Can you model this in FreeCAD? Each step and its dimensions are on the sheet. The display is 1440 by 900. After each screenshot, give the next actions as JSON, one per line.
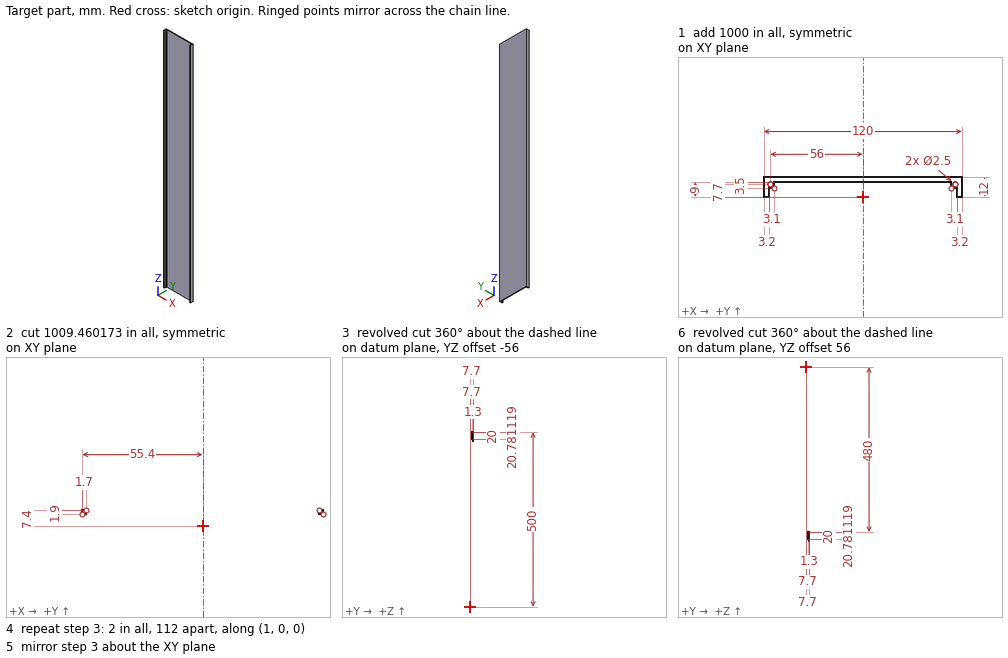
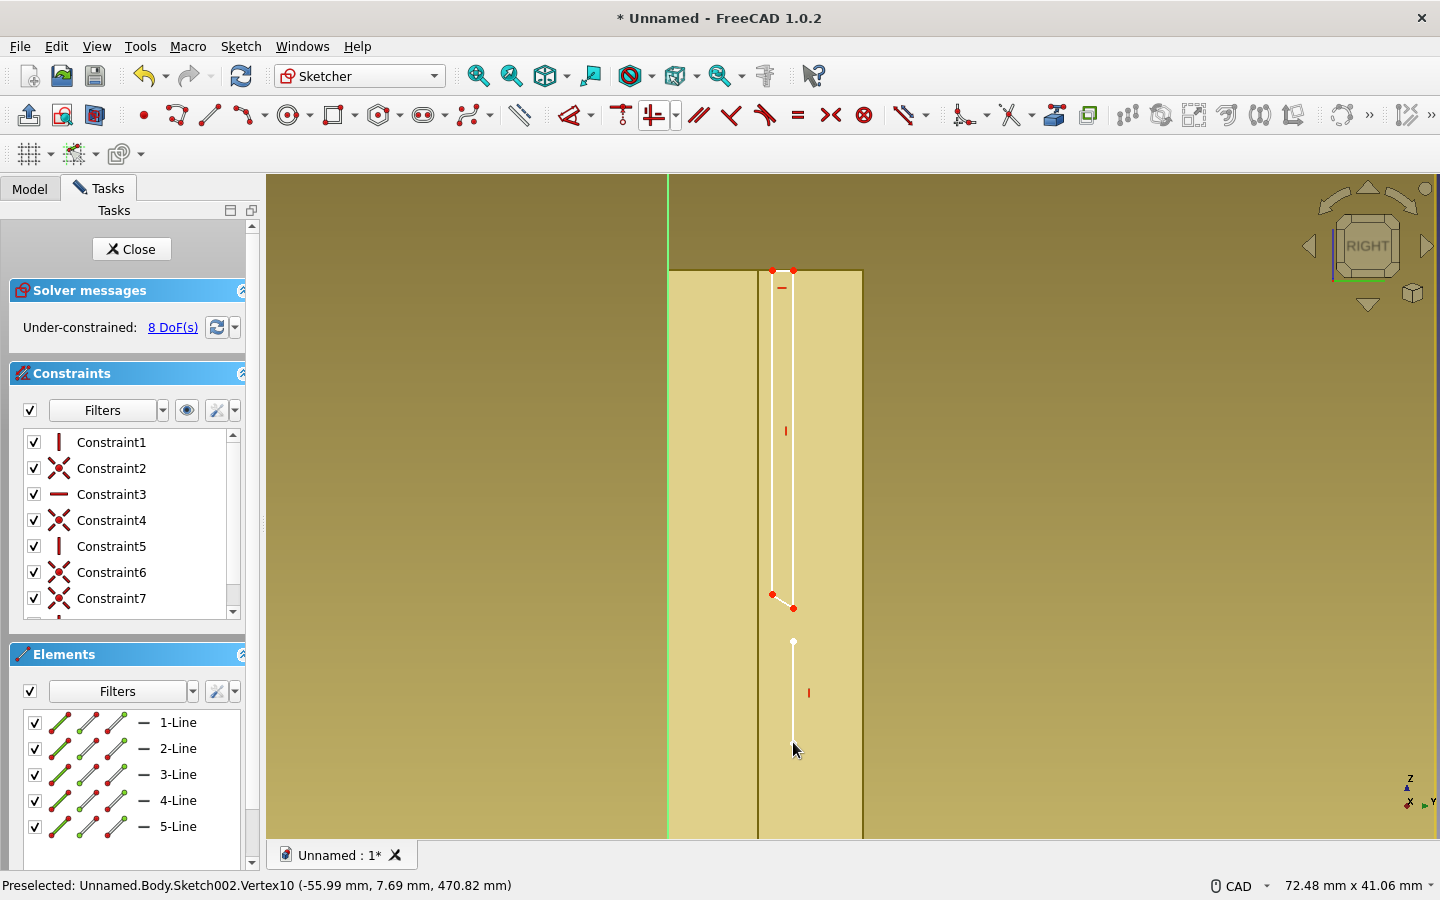
{"action": "left_click", "coordinate": [793, 672]}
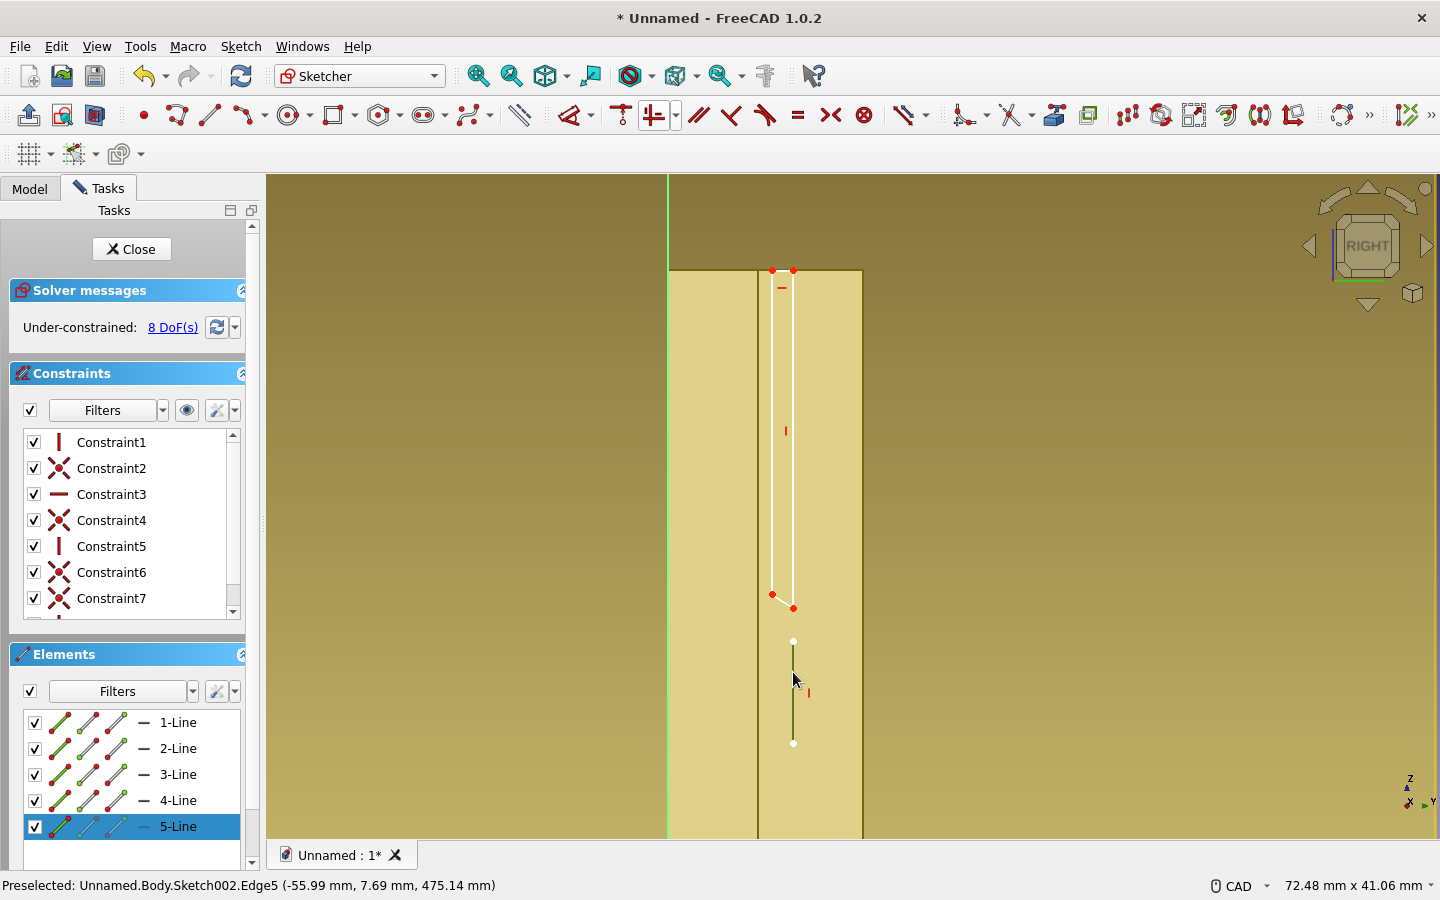
{"action": "key", "text": "g n"}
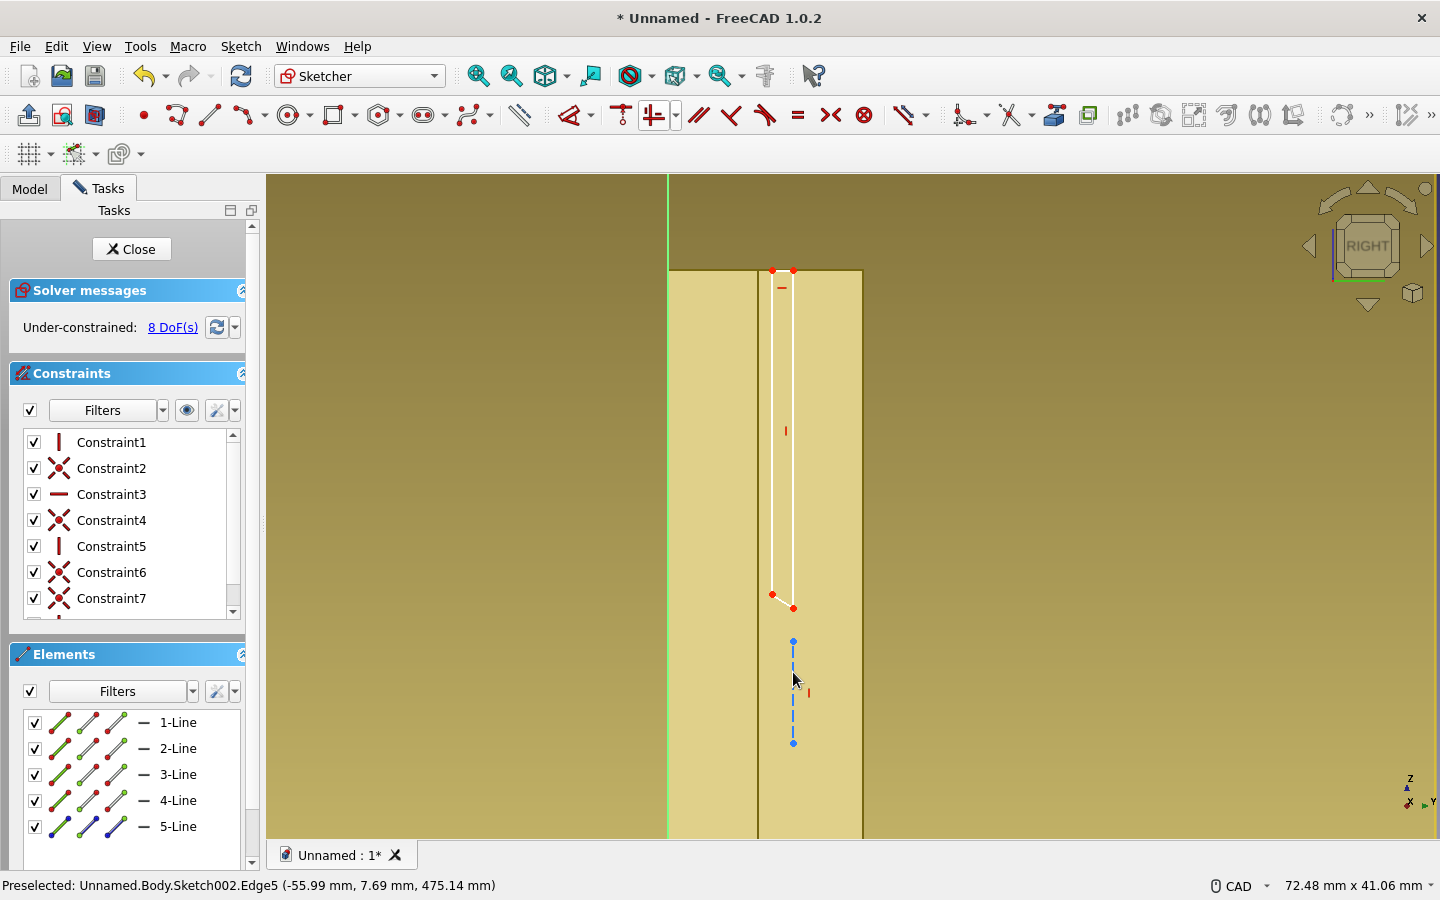
{"action": "left_click", "coordinate": [568, 116]}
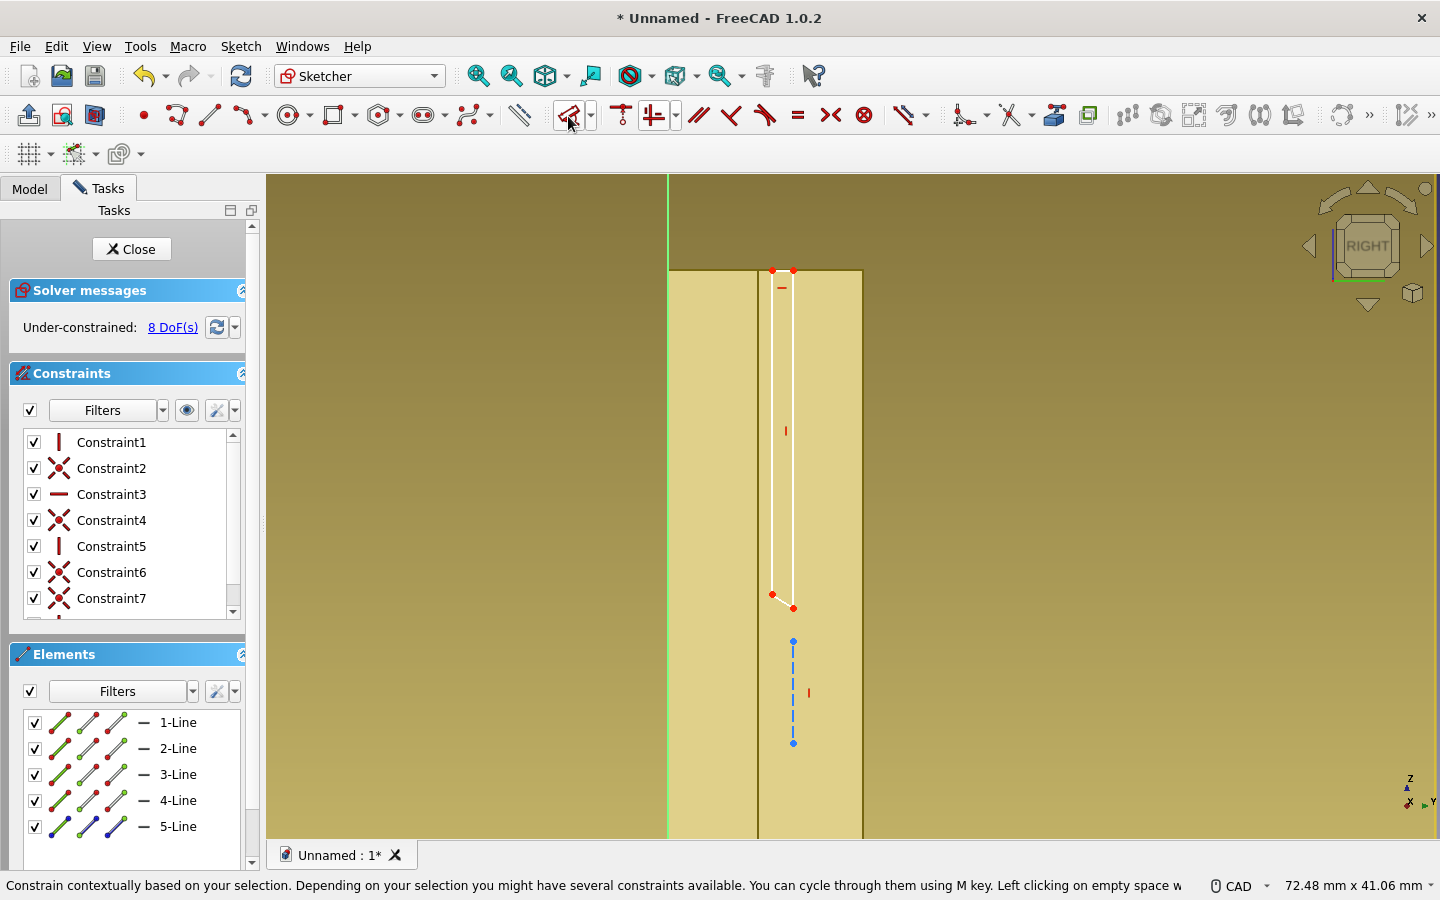
{"action": "left_click", "coordinate": [772, 368]}
{"action": "left_click", "coordinate": [738, 433]}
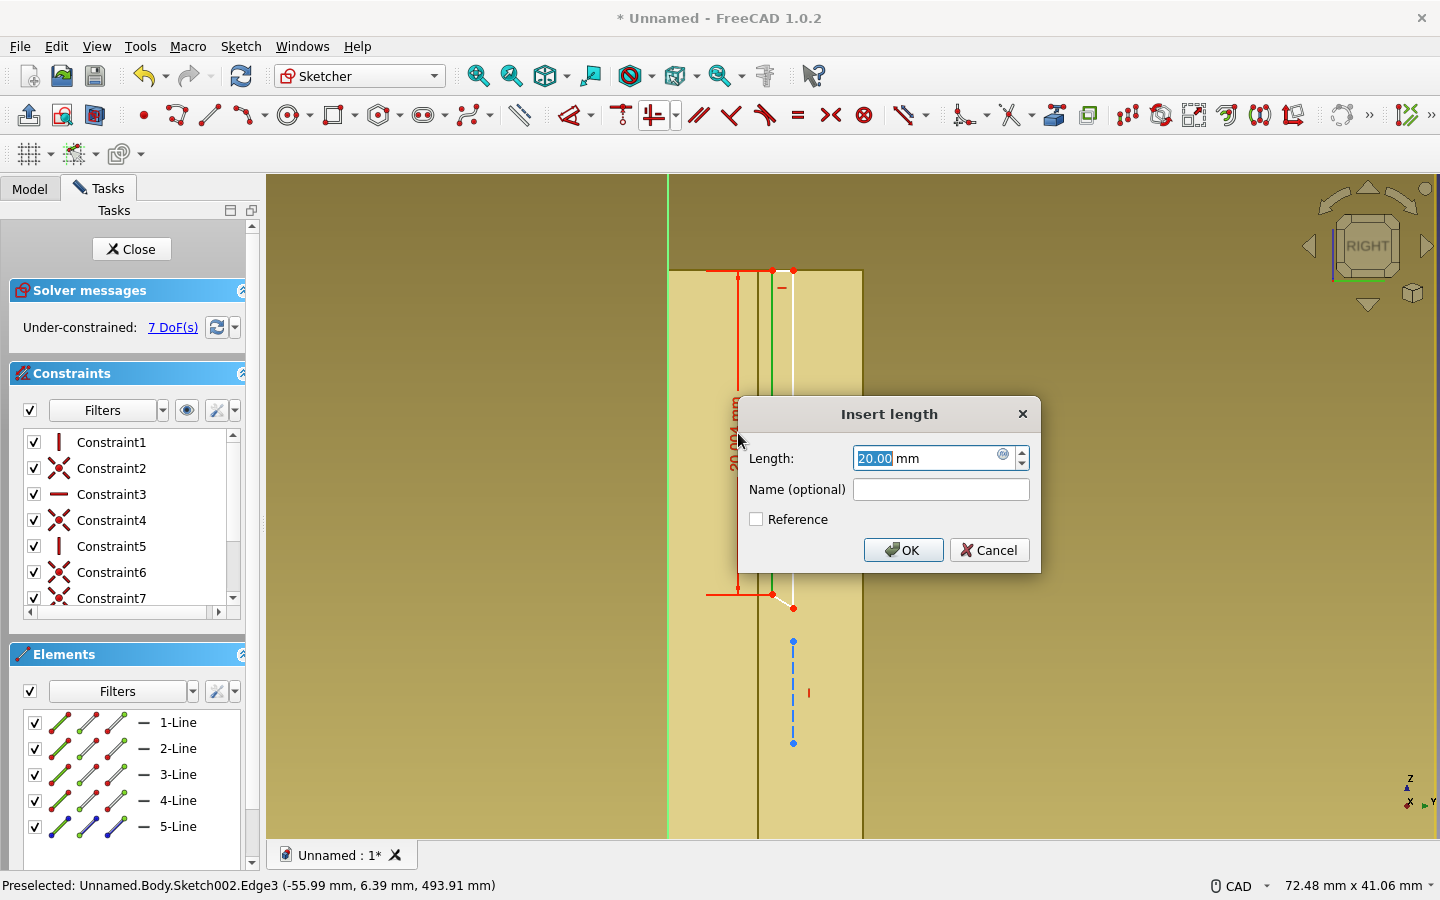
{"action": "type", "text": "20"}
{"action": "key", "text": "Return"}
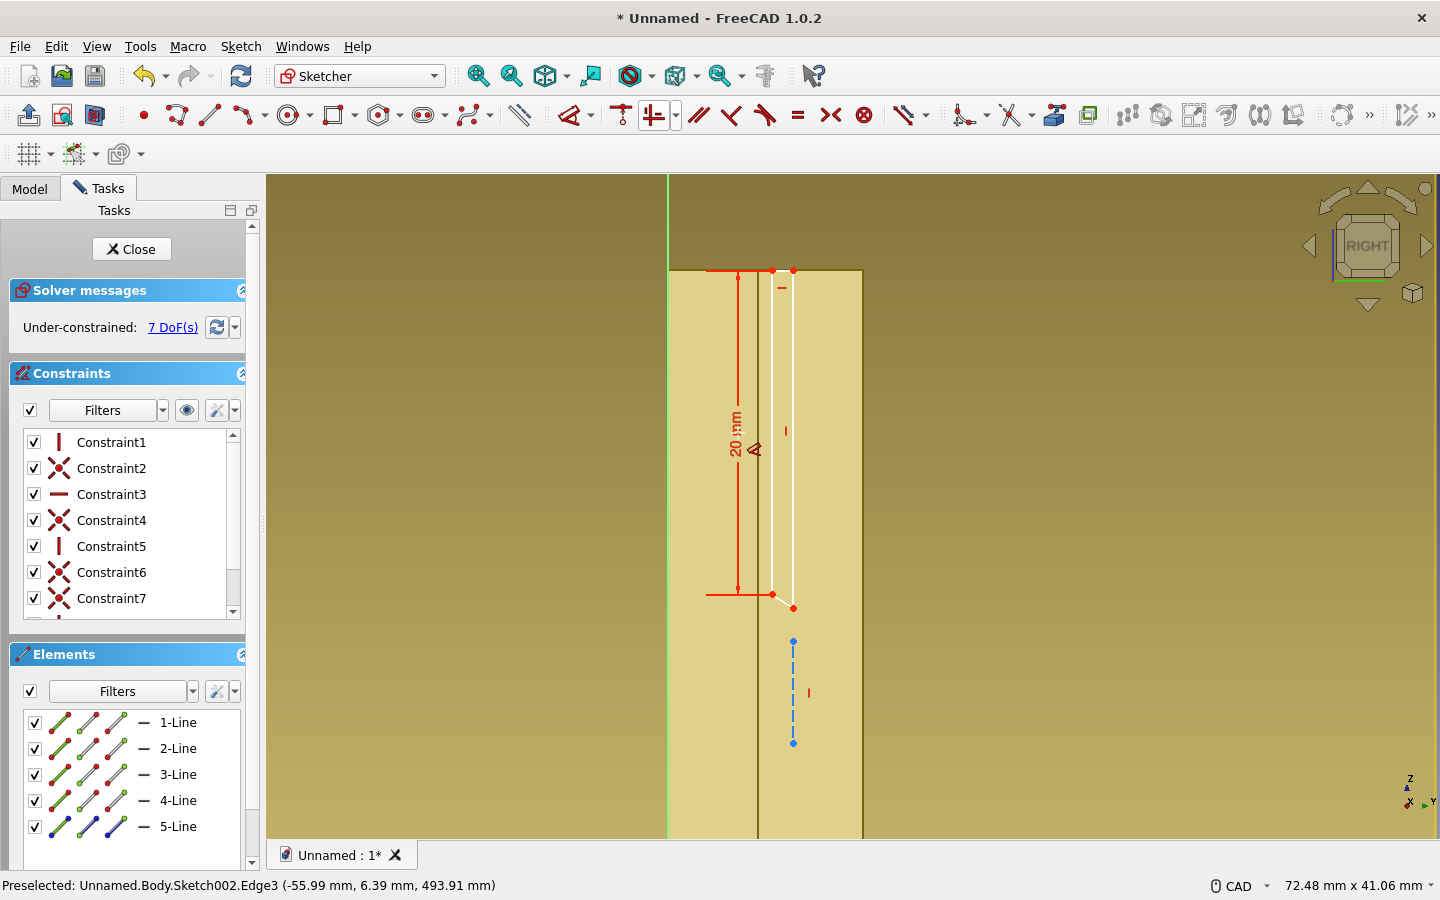
{"action": "scroll", "coordinate": [783, 271], "scroll_direction": "up", "scroll_amount": 4}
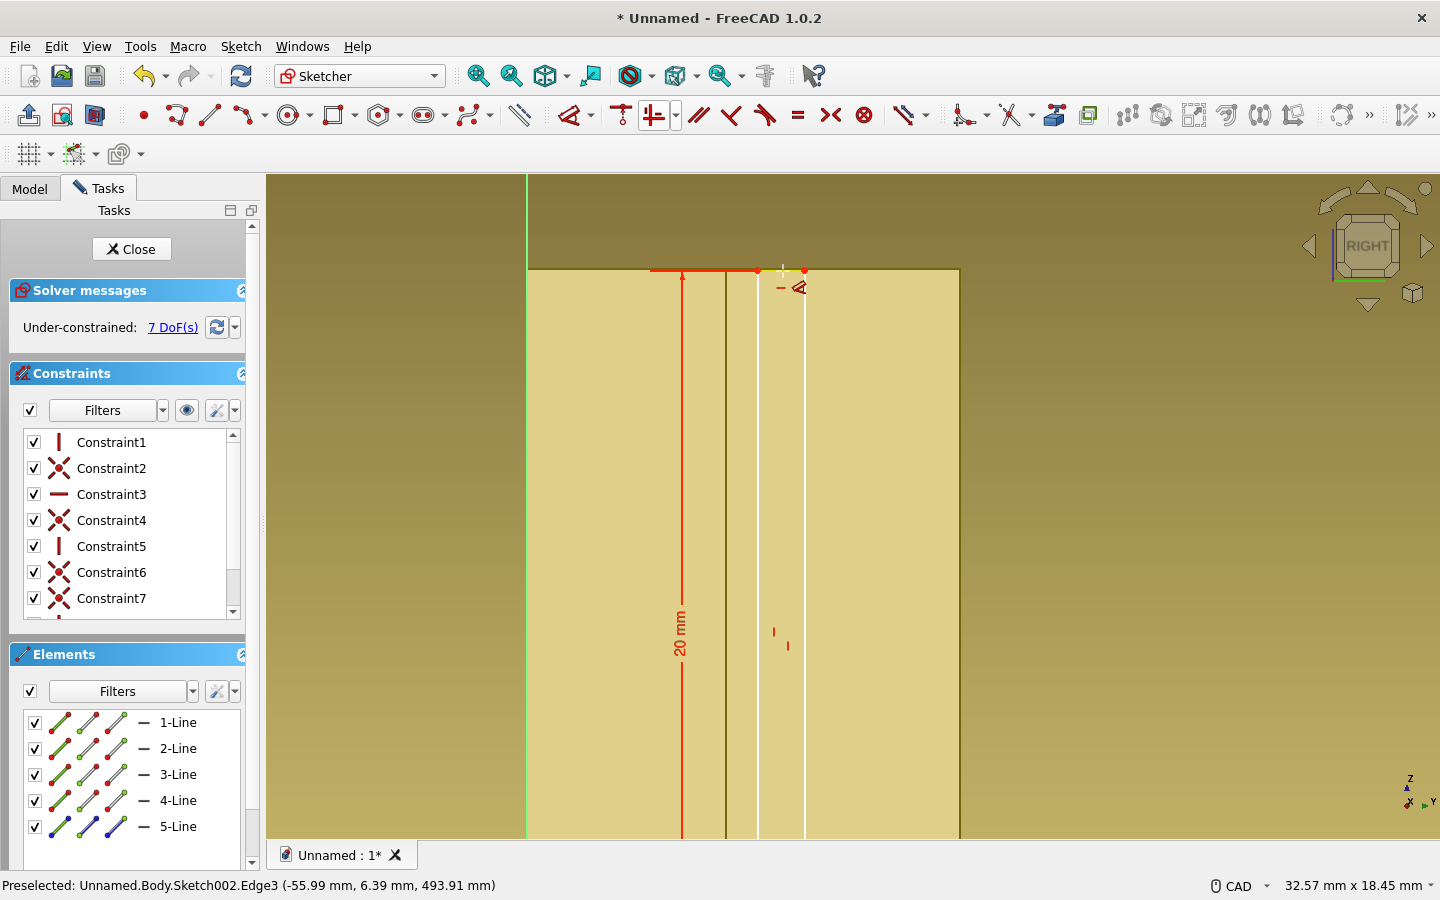
{"action": "left_click", "coordinate": [781, 271]}
{"action": "left_click", "coordinate": [781, 237]}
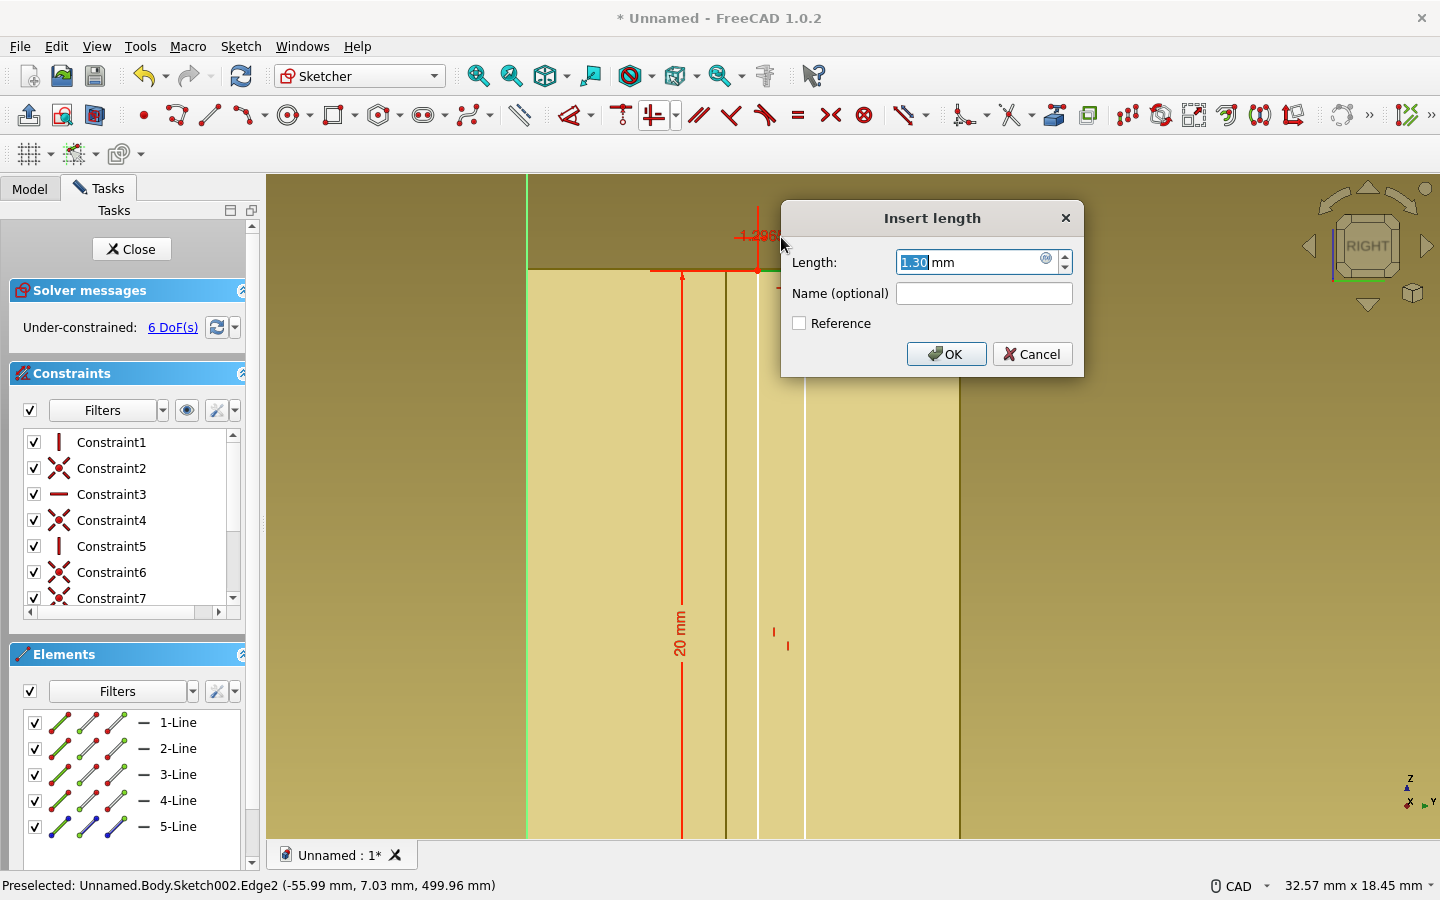
{"action": "type", "text": "1.3"}
{"action": "key", "text": "Return"}